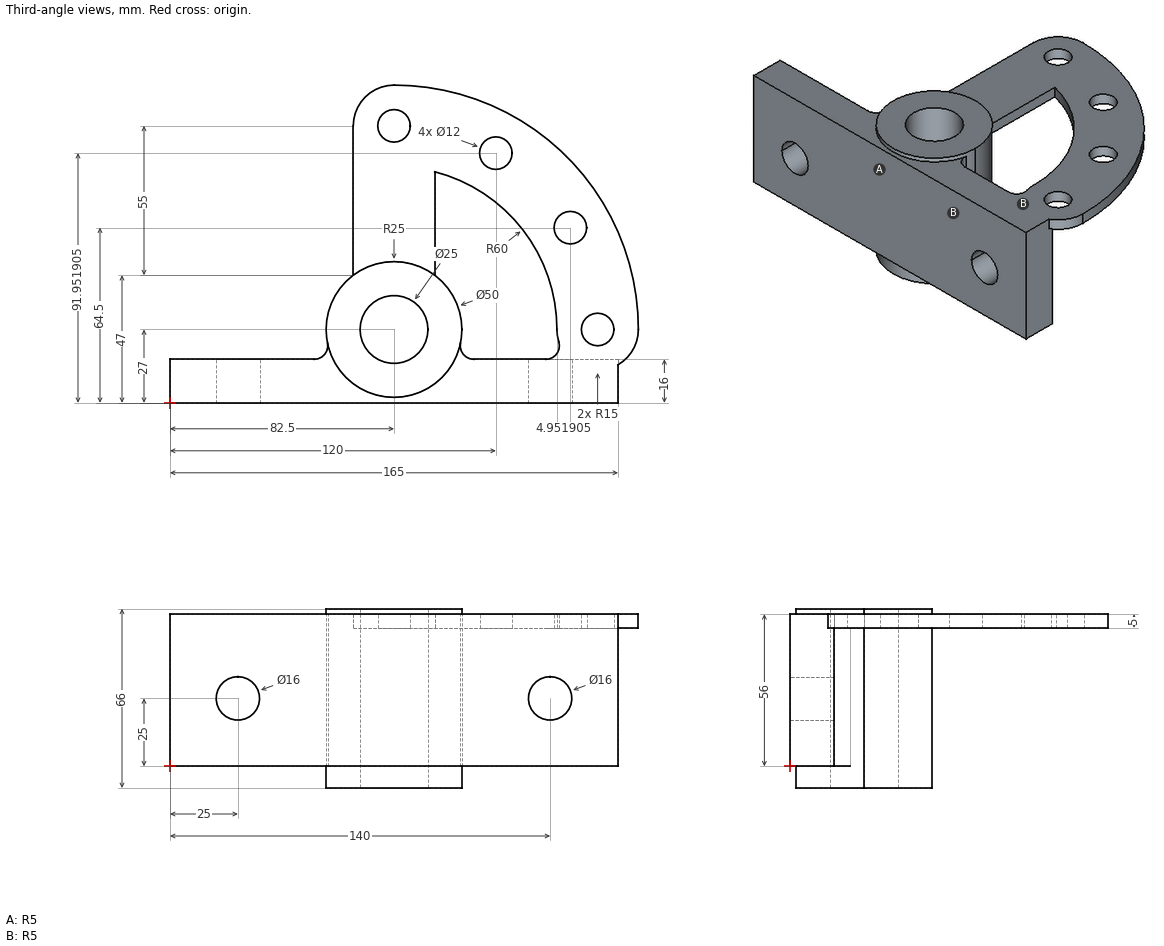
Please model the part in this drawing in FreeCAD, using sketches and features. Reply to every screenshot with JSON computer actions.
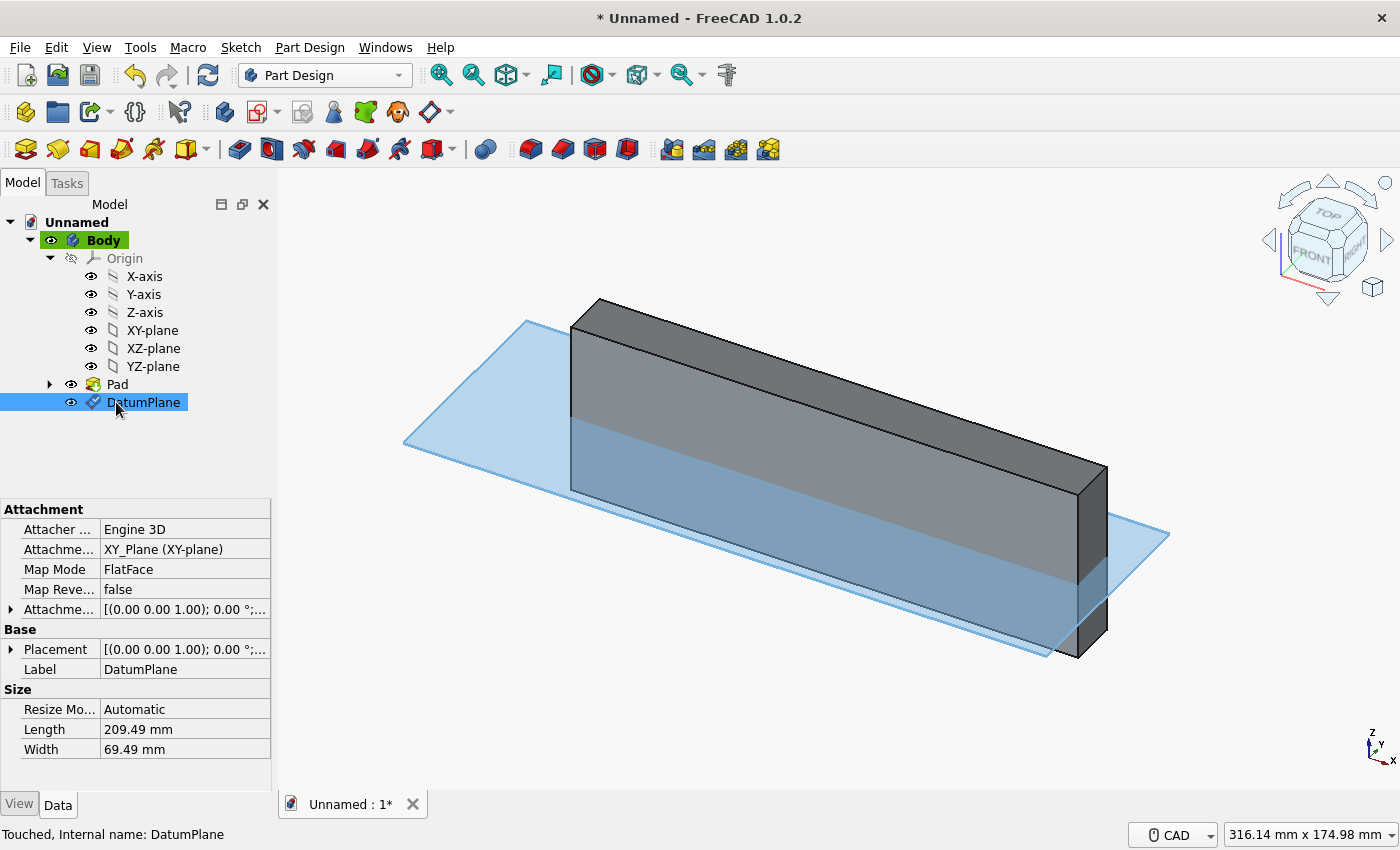
{"action": "left_click", "coordinate": [258, 112]}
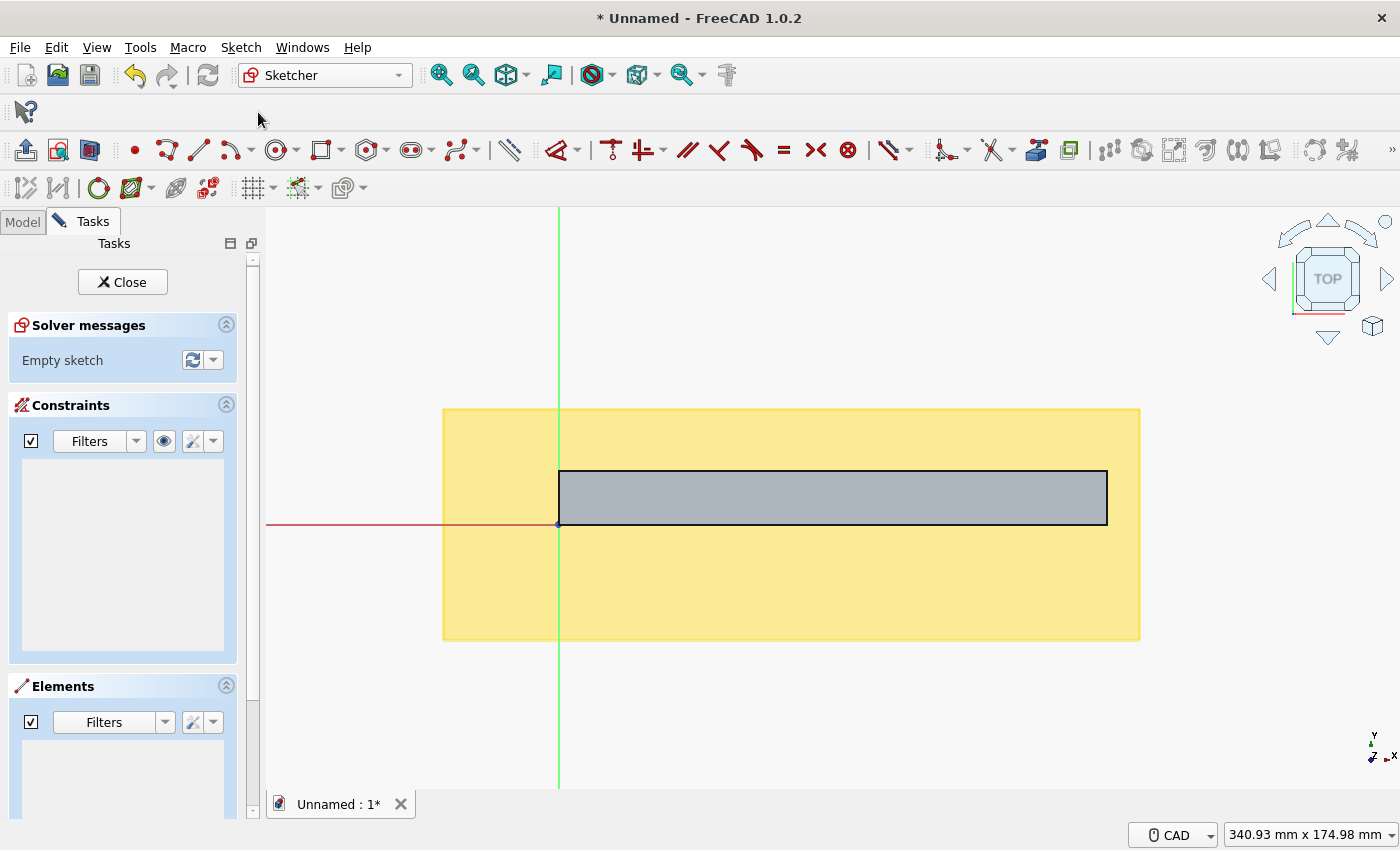
{"action": "left_click", "coordinate": [90, 150]}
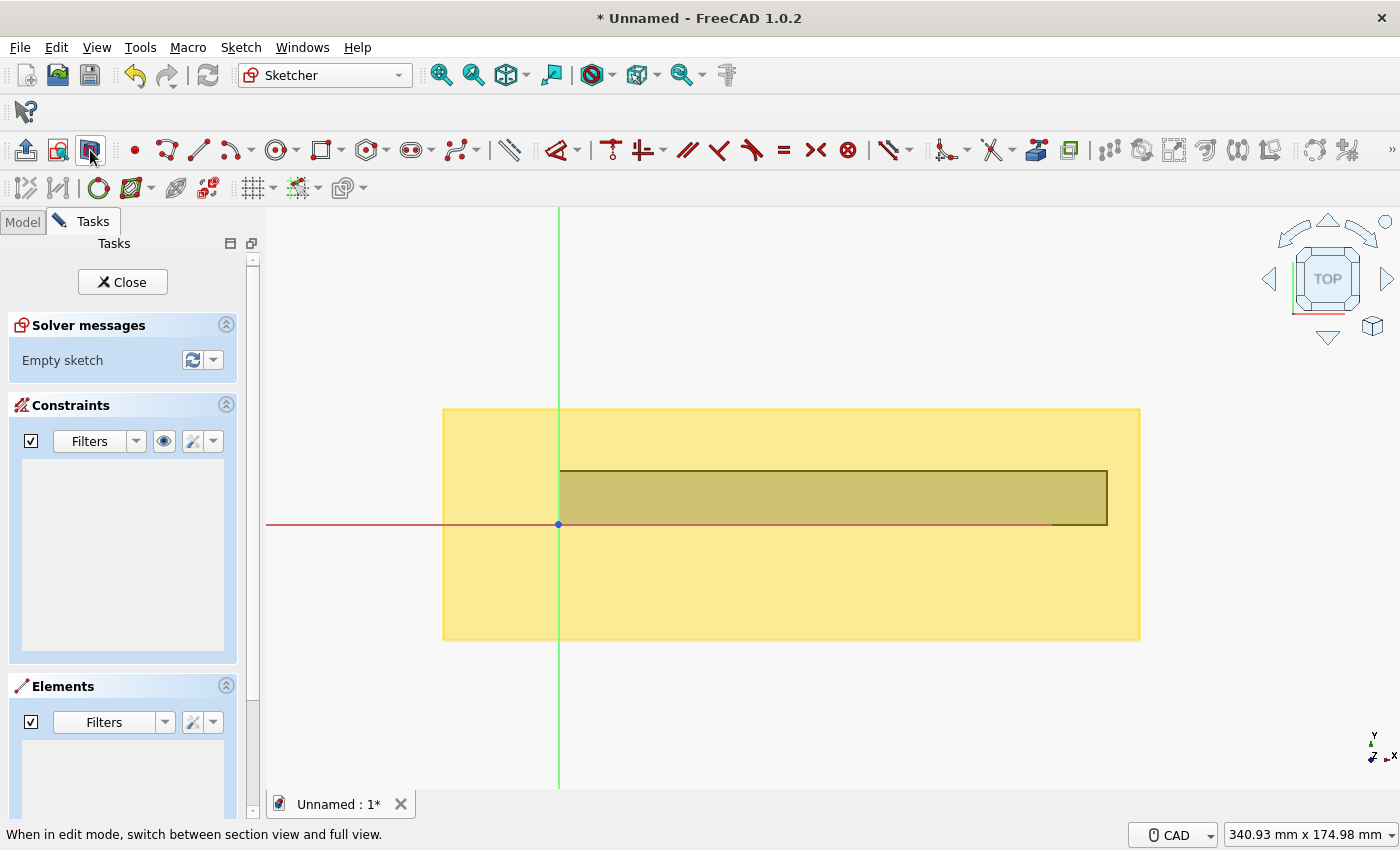
{"action": "scroll", "coordinate": [704, 365], "scroll_direction": "up", "scroll_amount": 3}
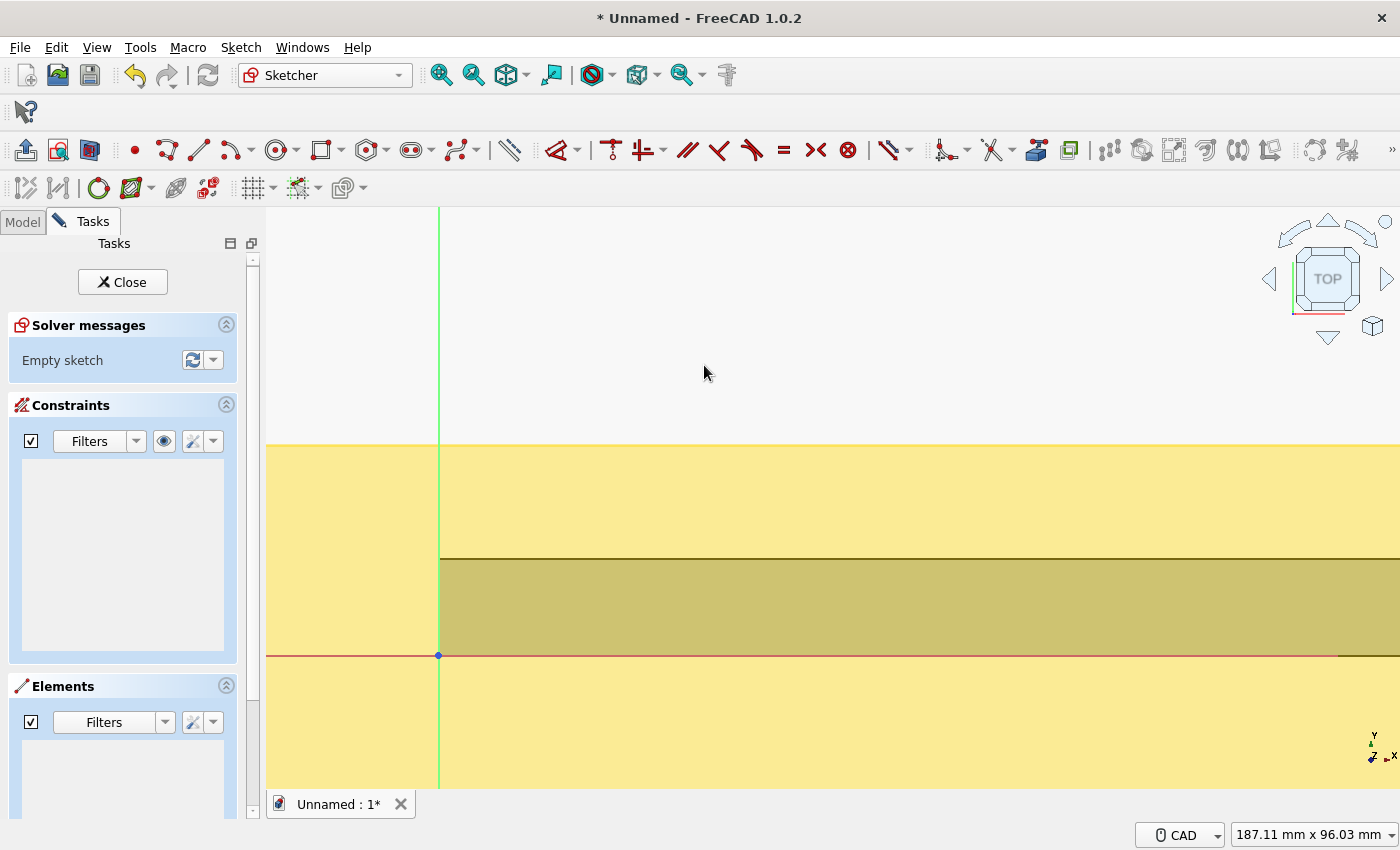
{"action": "left_click", "coordinate": [276, 150]}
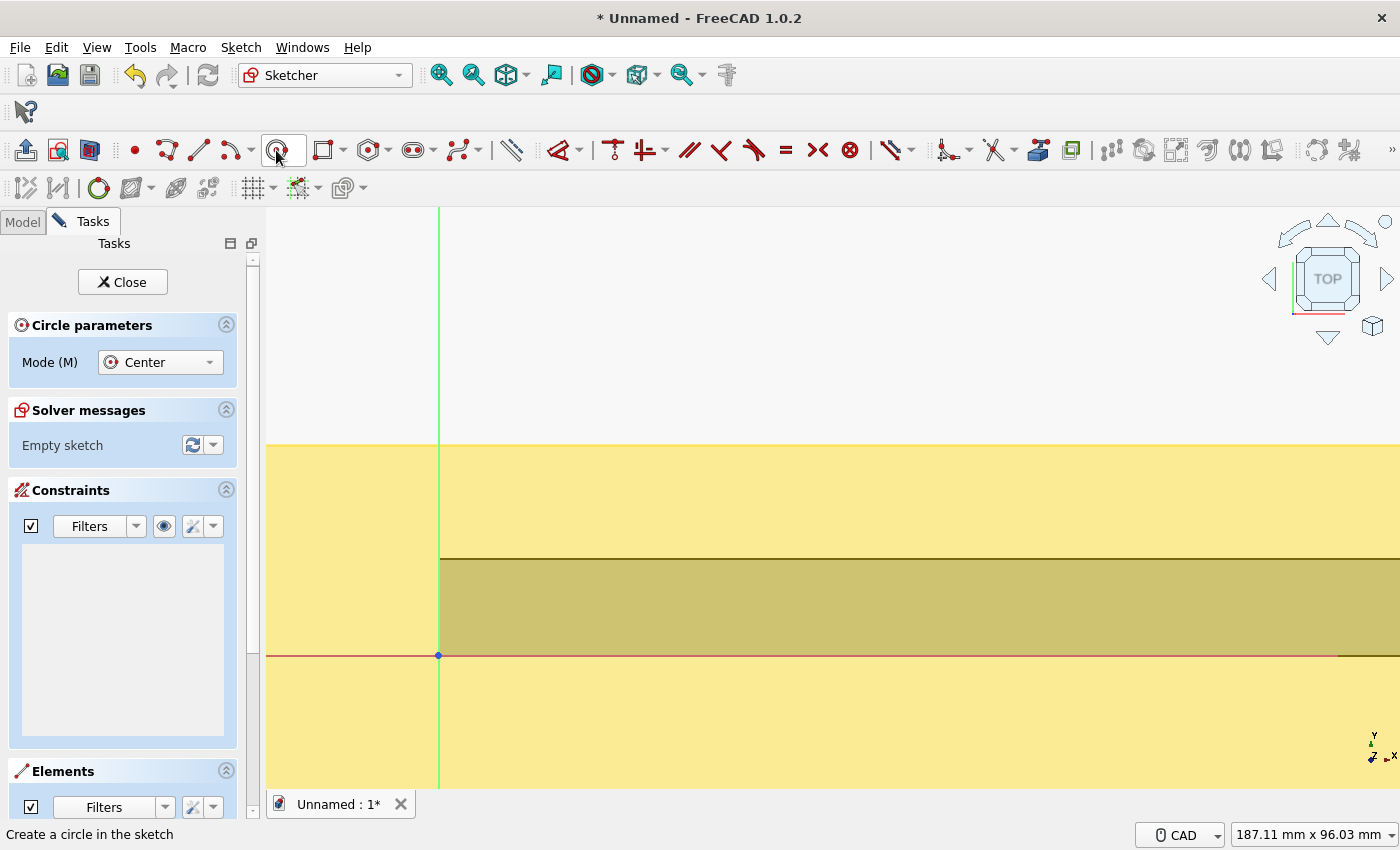
{"action": "left_click", "coordinate": [939, 492]}
{"action": "left_click", "coordinate": [1046, 385]}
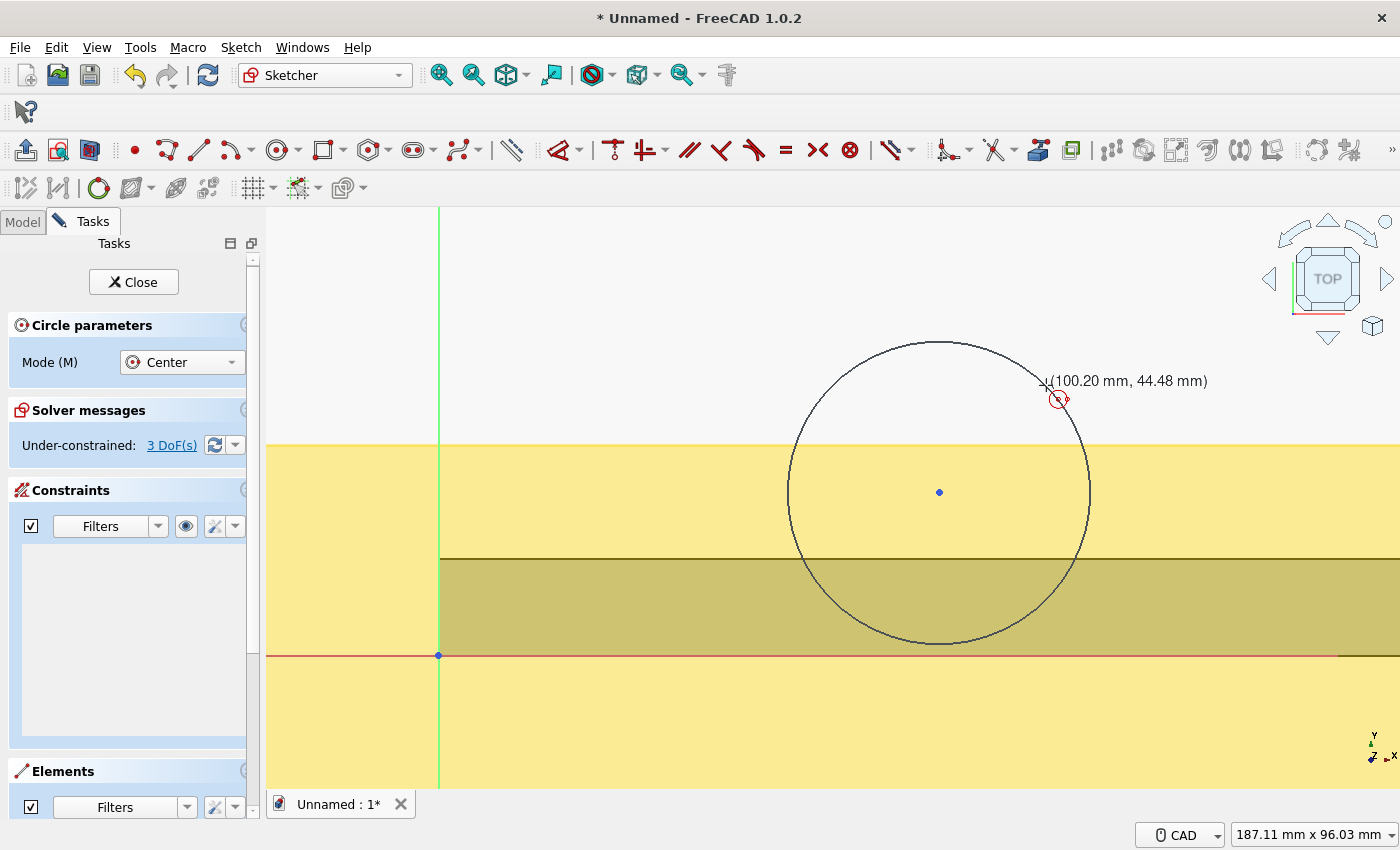
{"action": "left_click", "coordinate": [939, 493]}
{"action": "left_click", "coordinate": [992, 438]}
{"action": "key", "text": "Escape"}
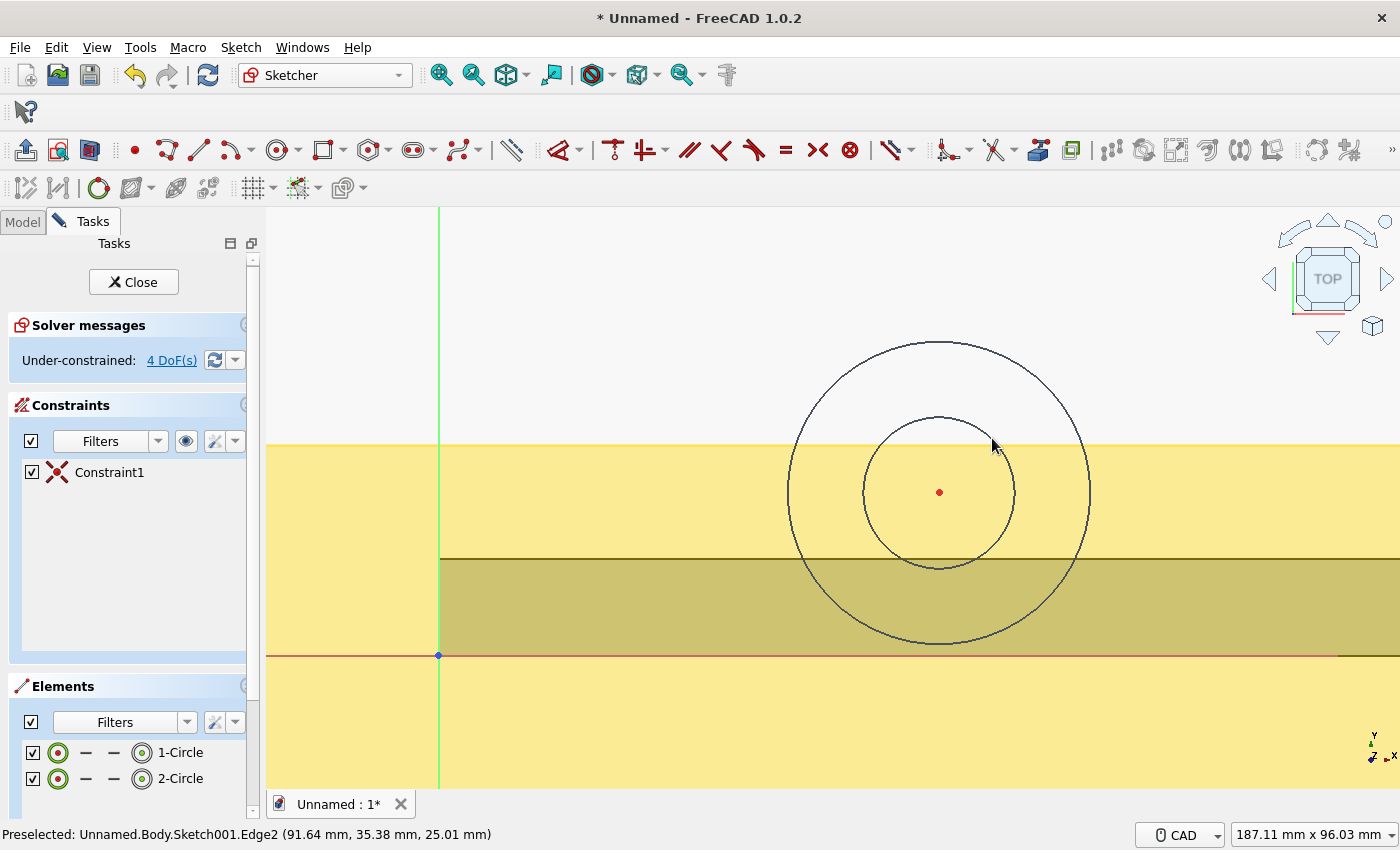
{"action": "left_click", "coordinate": [558, 150]}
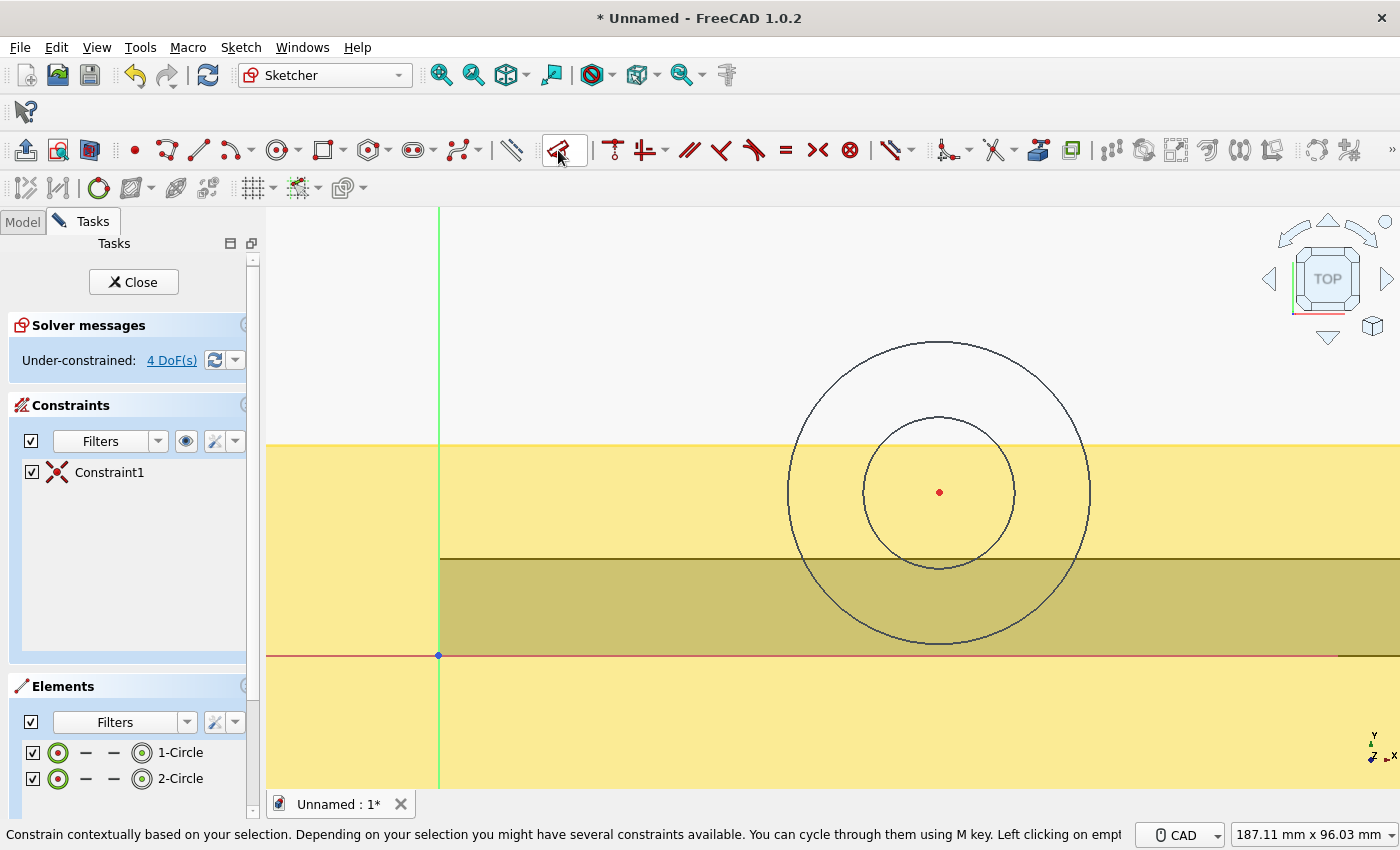
{"action": "left_click", "coordinate": [1046, 386]}
{"action": "left_click", "coordinate": [1069, 363]}